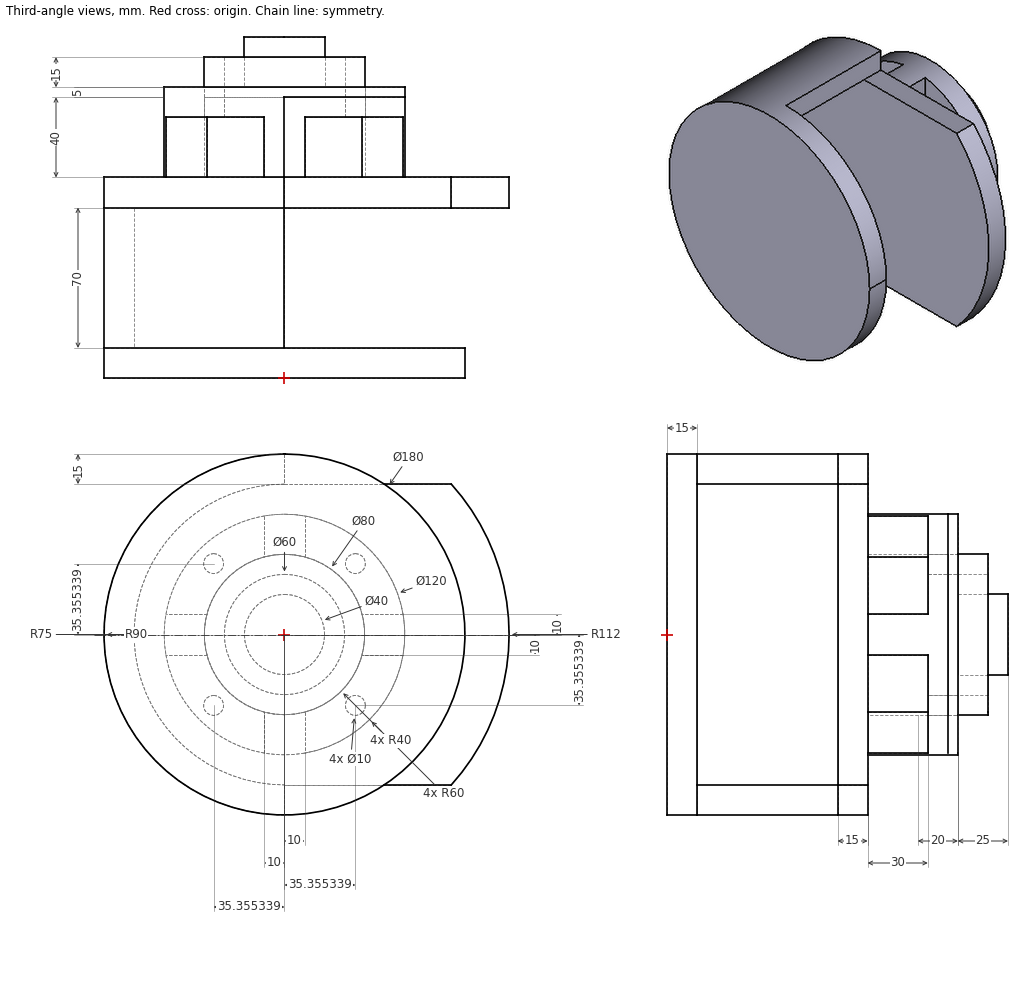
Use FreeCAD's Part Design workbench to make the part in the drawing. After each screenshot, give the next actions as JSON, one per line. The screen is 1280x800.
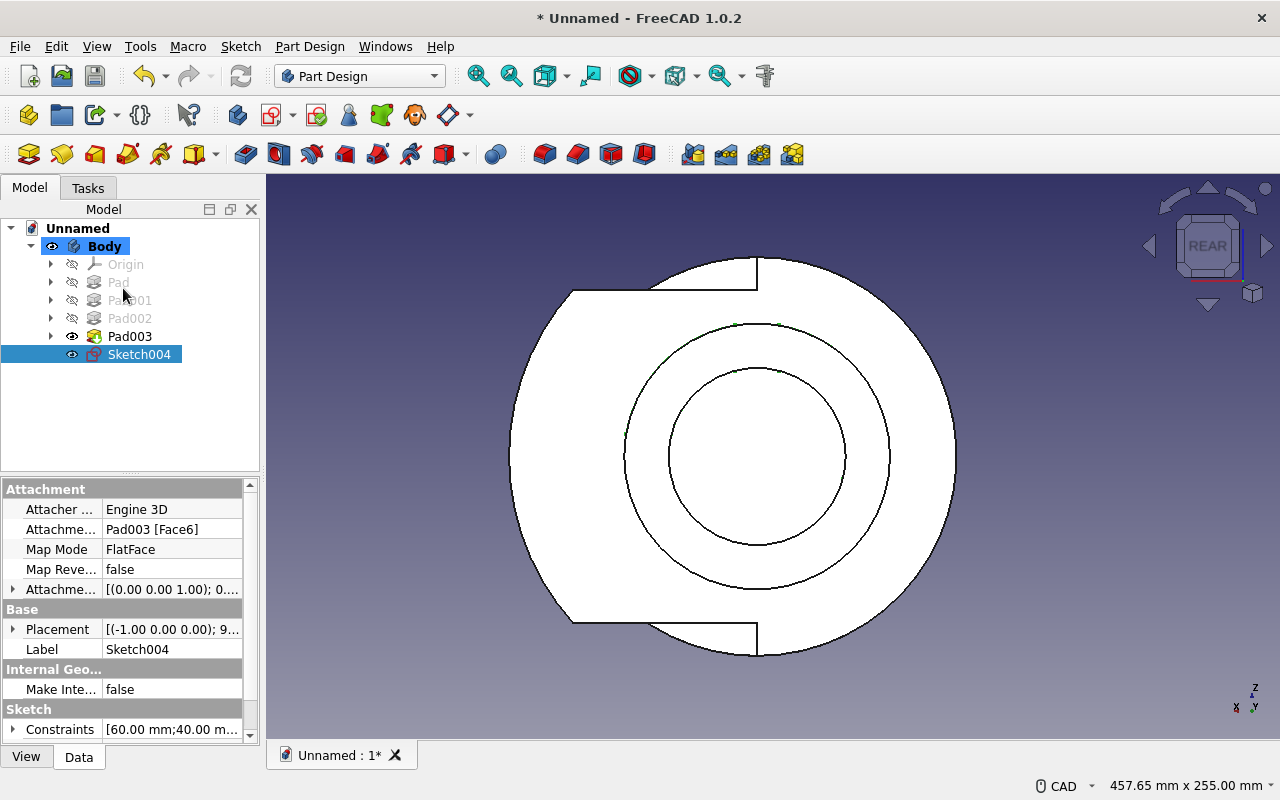
{"action": "left_click", "coordinate": [246, 154]}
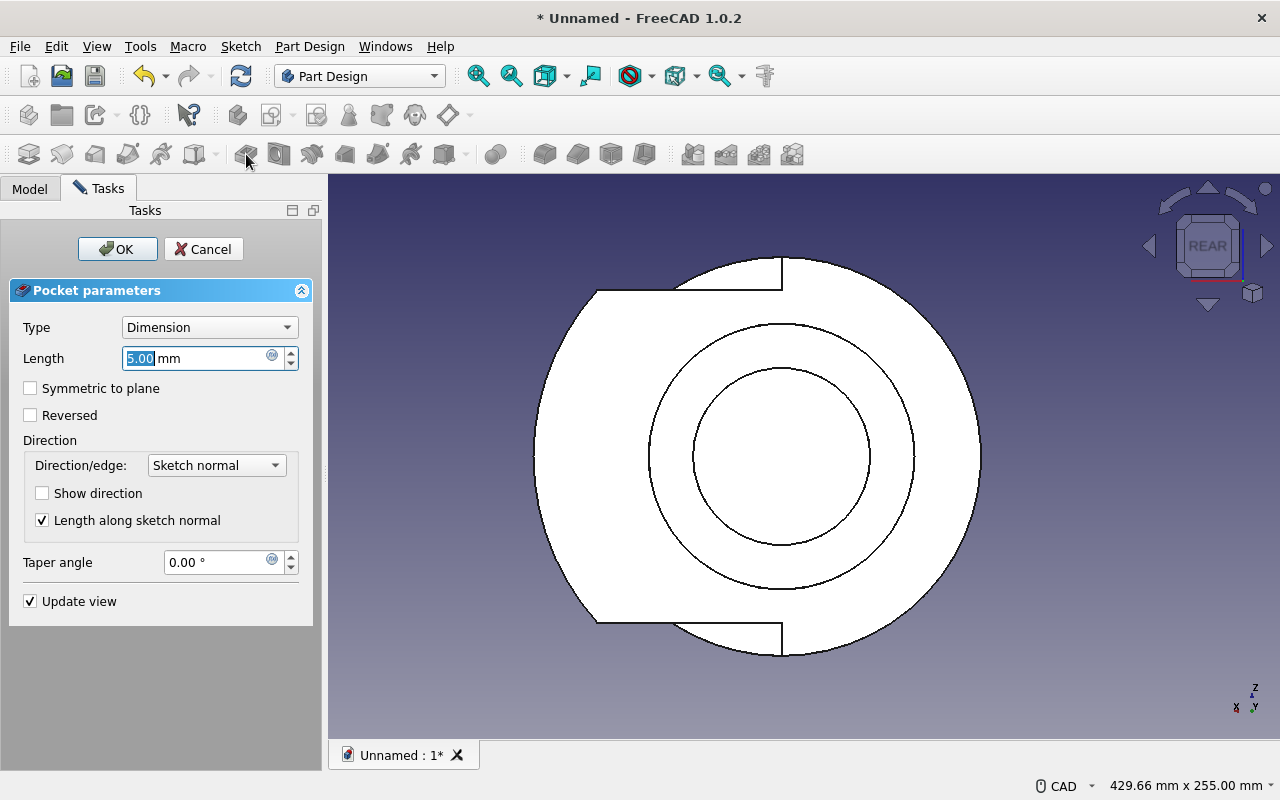
{"action": "type", "text": "30"}
{"action": "key", "text": "Tab"}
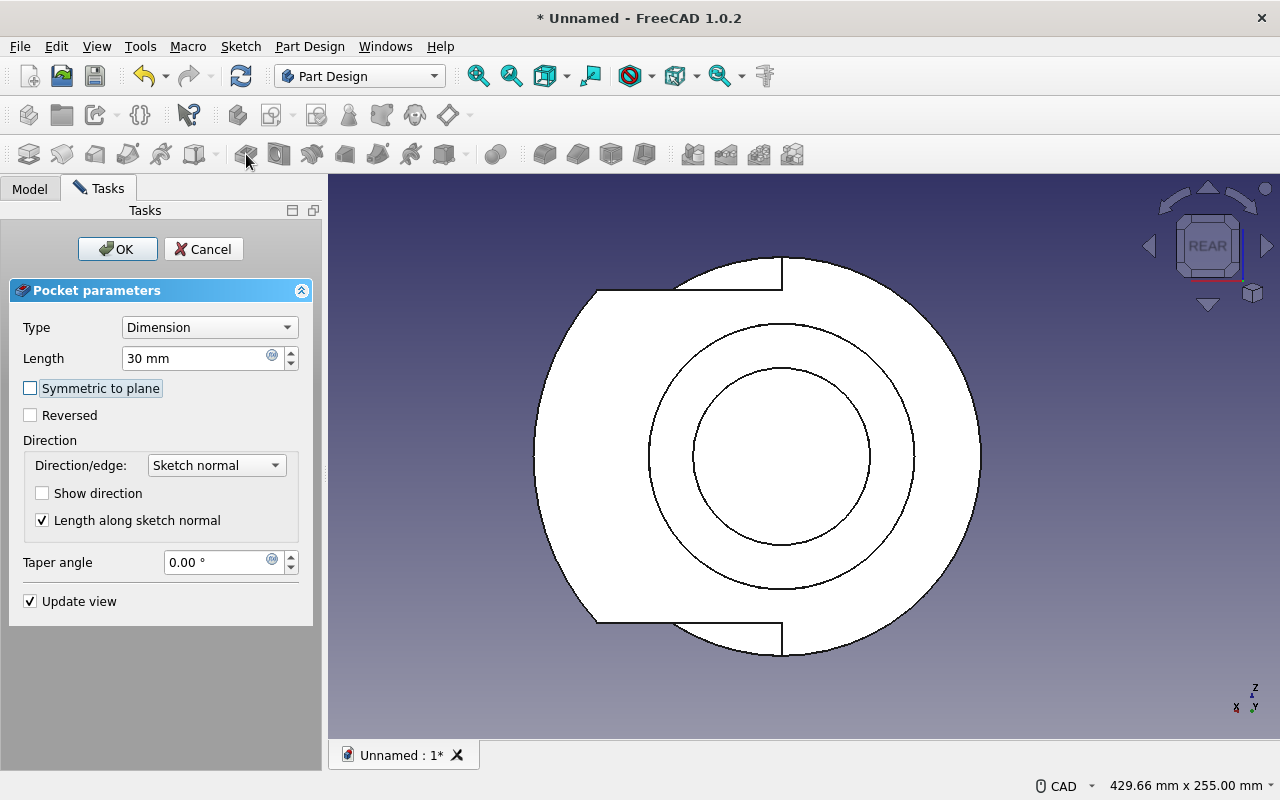
{"action": "left_click", "coordinate": [31, 415]}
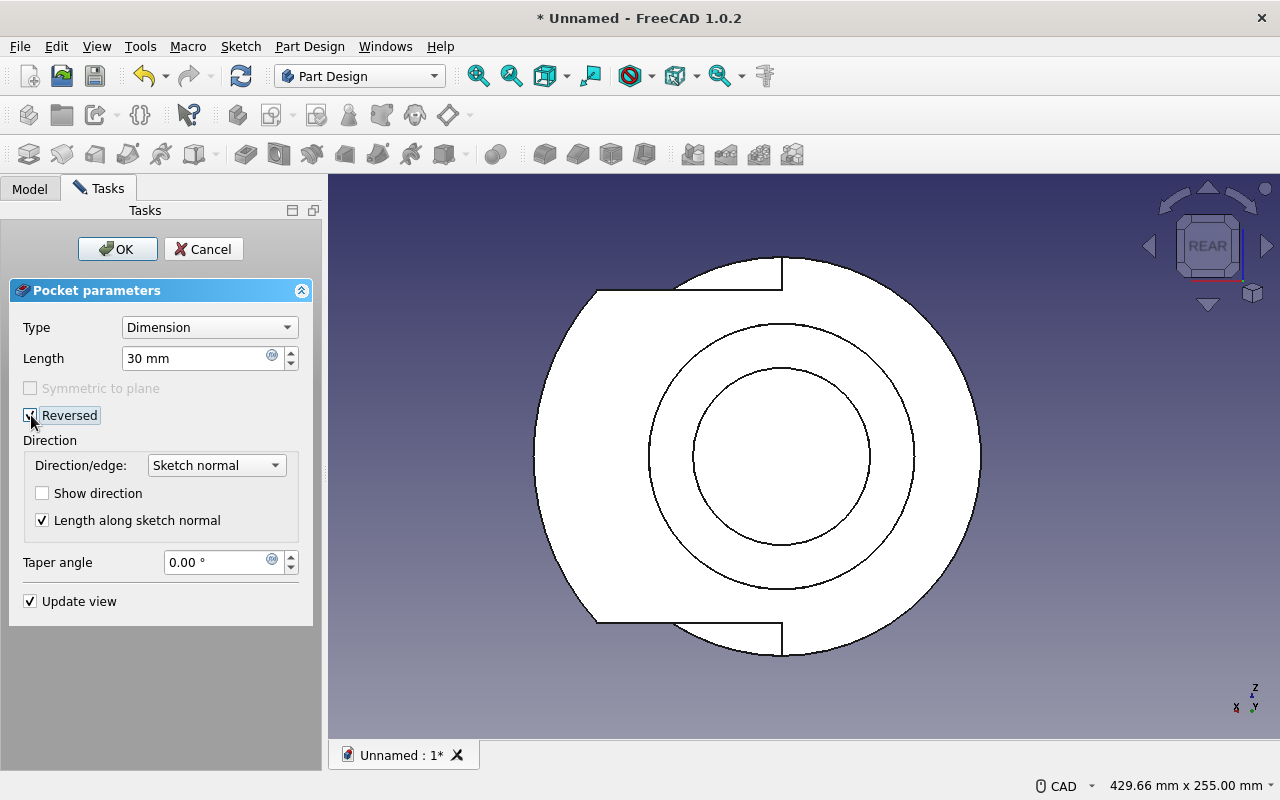
{"action": "left_click", "coordinate": [118, 249]}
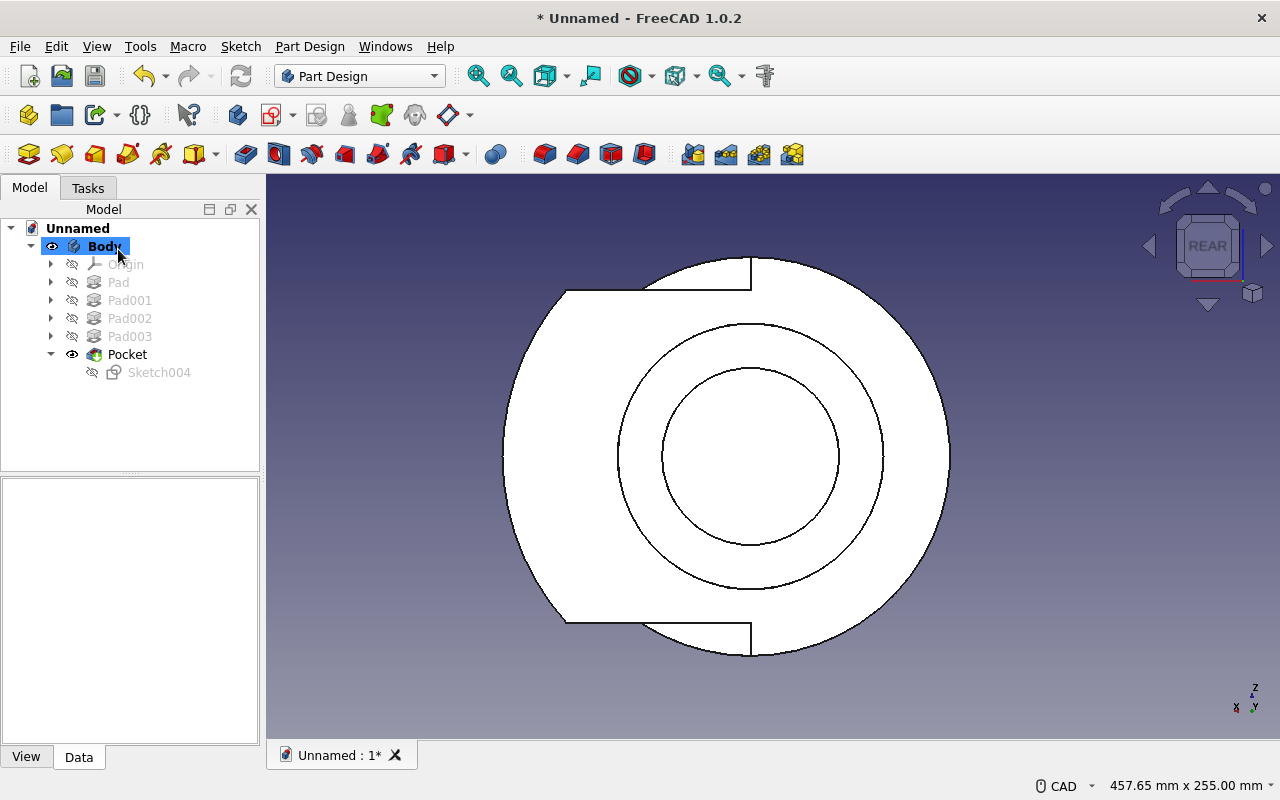
{"action": "left_click", "coordinate": [637, 455]}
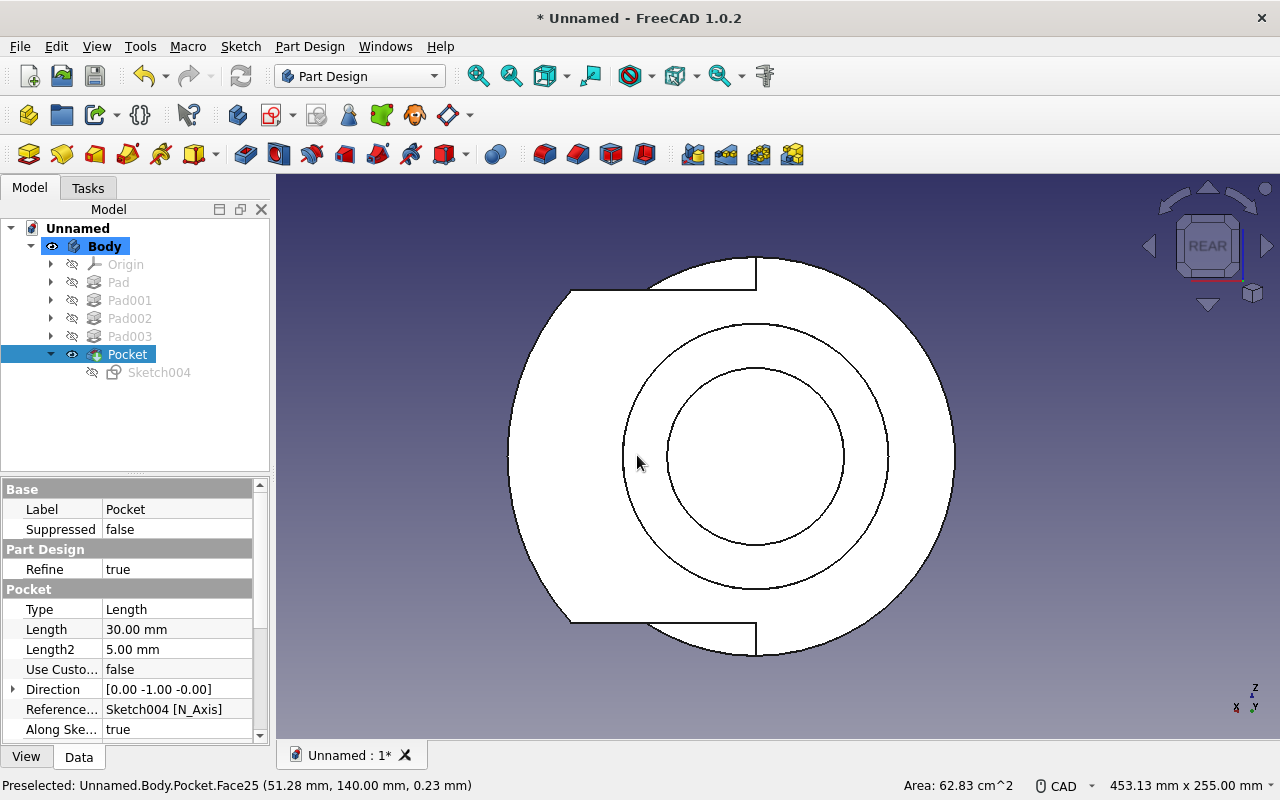
{"action": "left_click", "coordinate": [270, 116]}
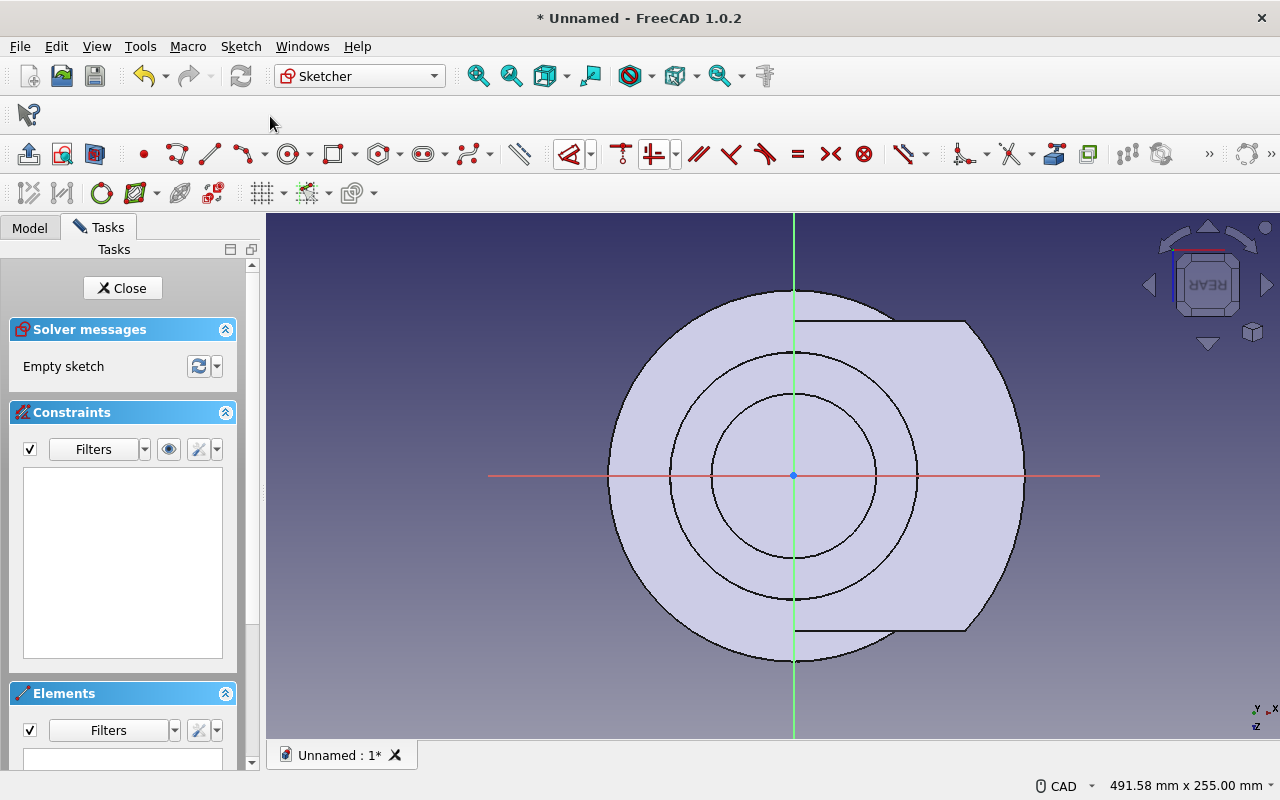
{"action": "left_click", "coordinate": [288, 154]}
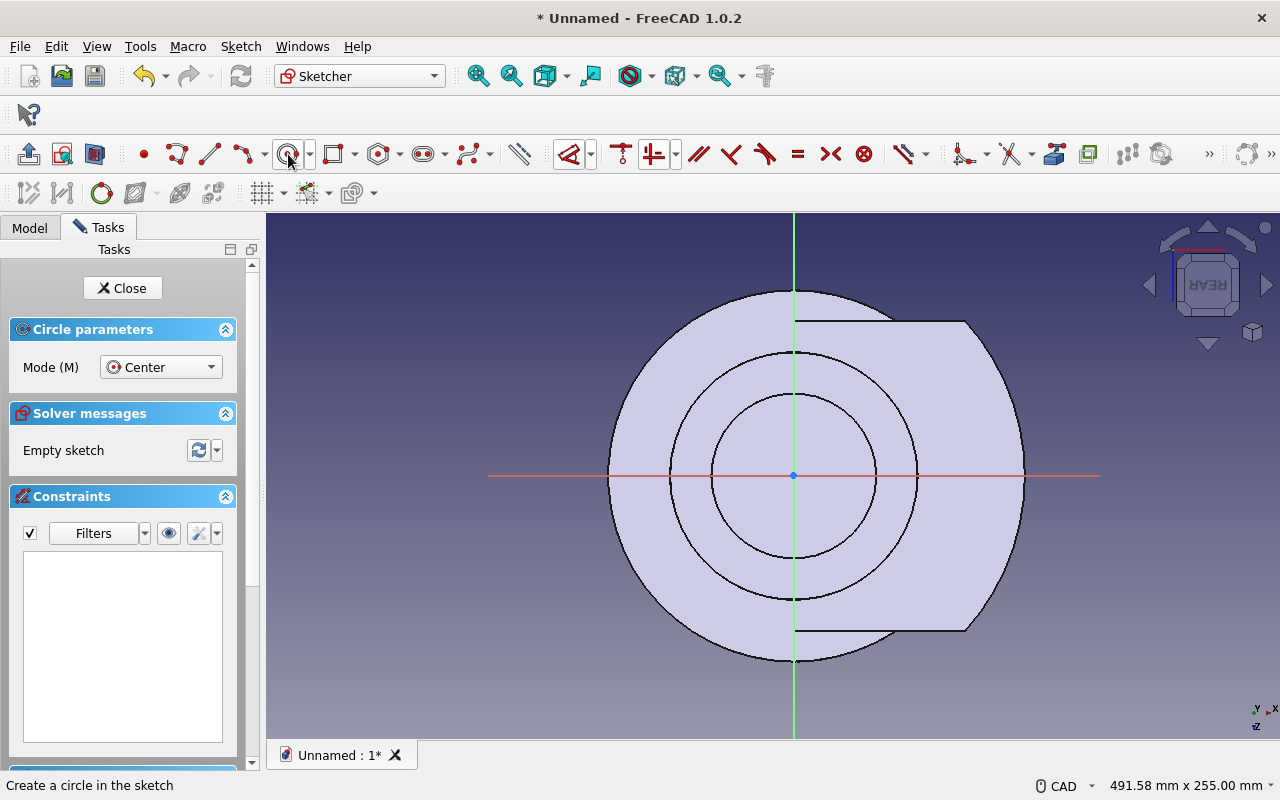
{"action": "left_click", "coordinate": [794, 476]}
{"action": "left_click", "coordinate": [881, 388]}
{"action": "key", "text": "Escape"}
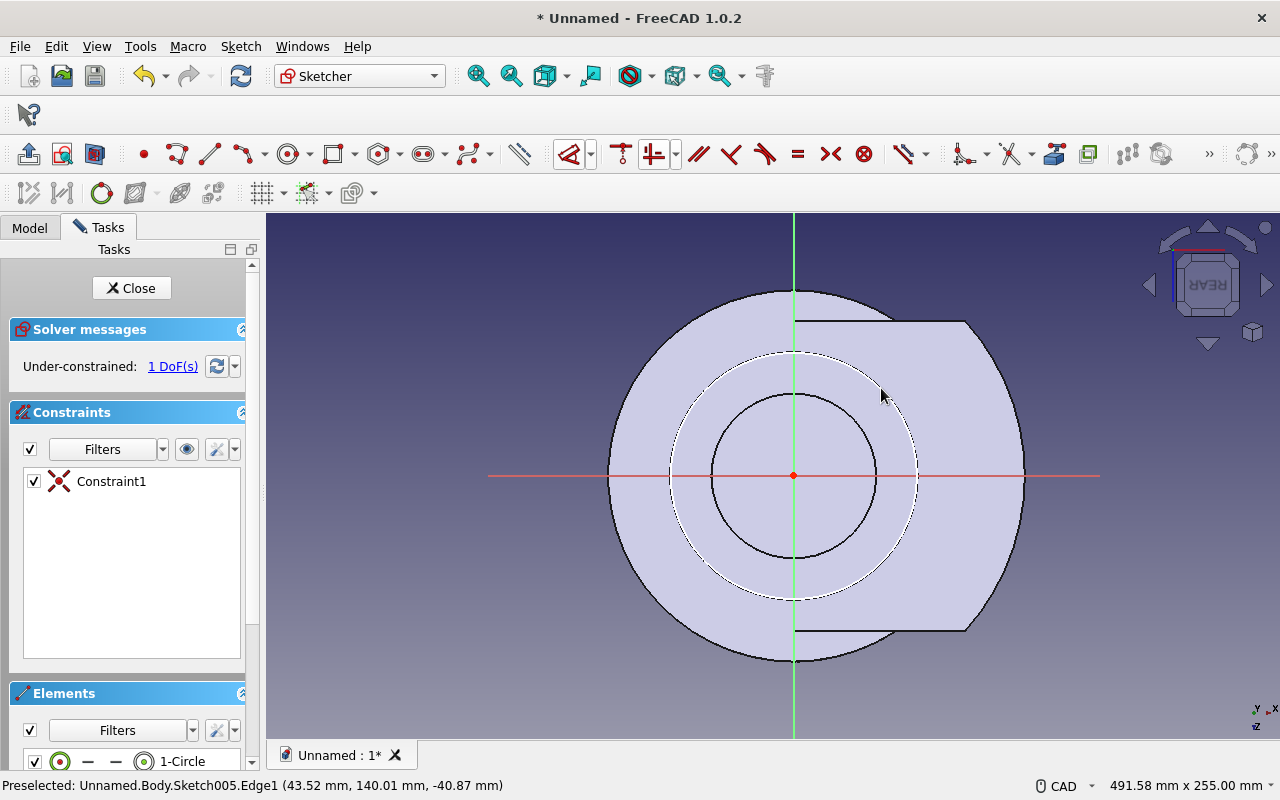
{"action": "left_click", "coordinate": [881, 389]}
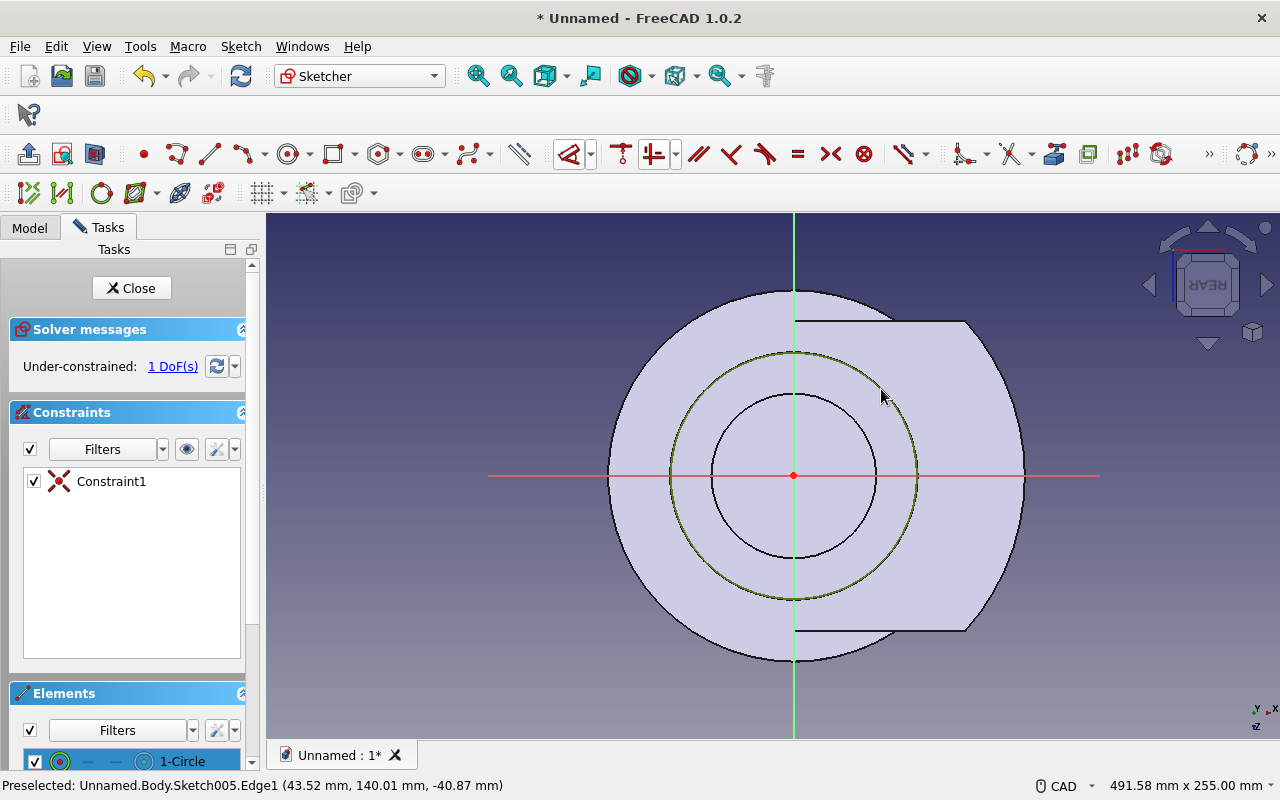
{"action": "key", "text": "k o"}